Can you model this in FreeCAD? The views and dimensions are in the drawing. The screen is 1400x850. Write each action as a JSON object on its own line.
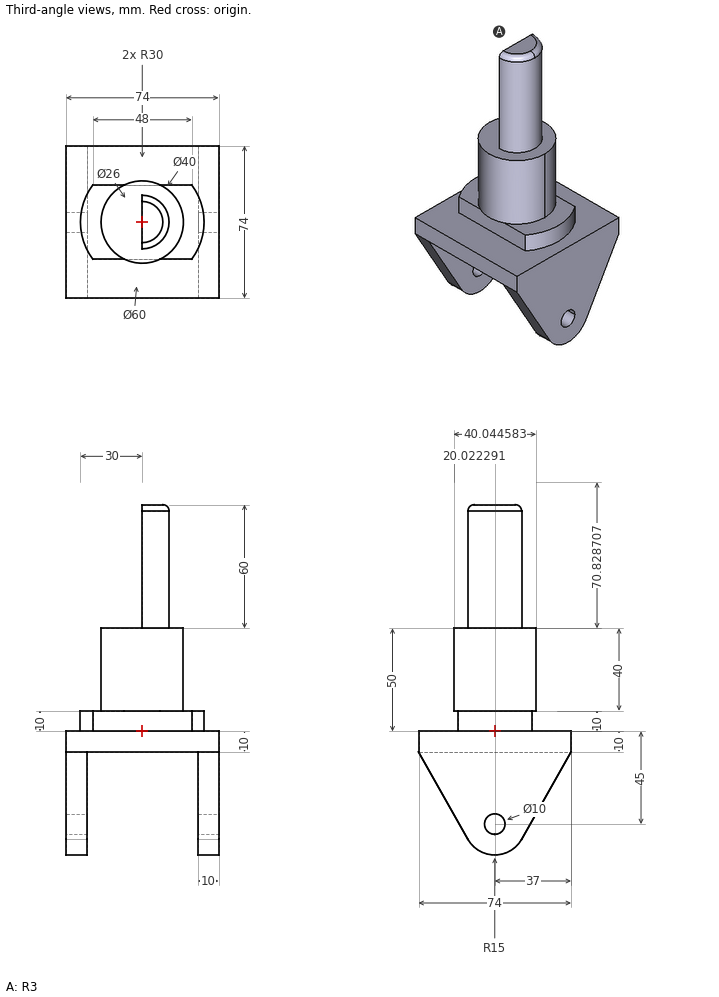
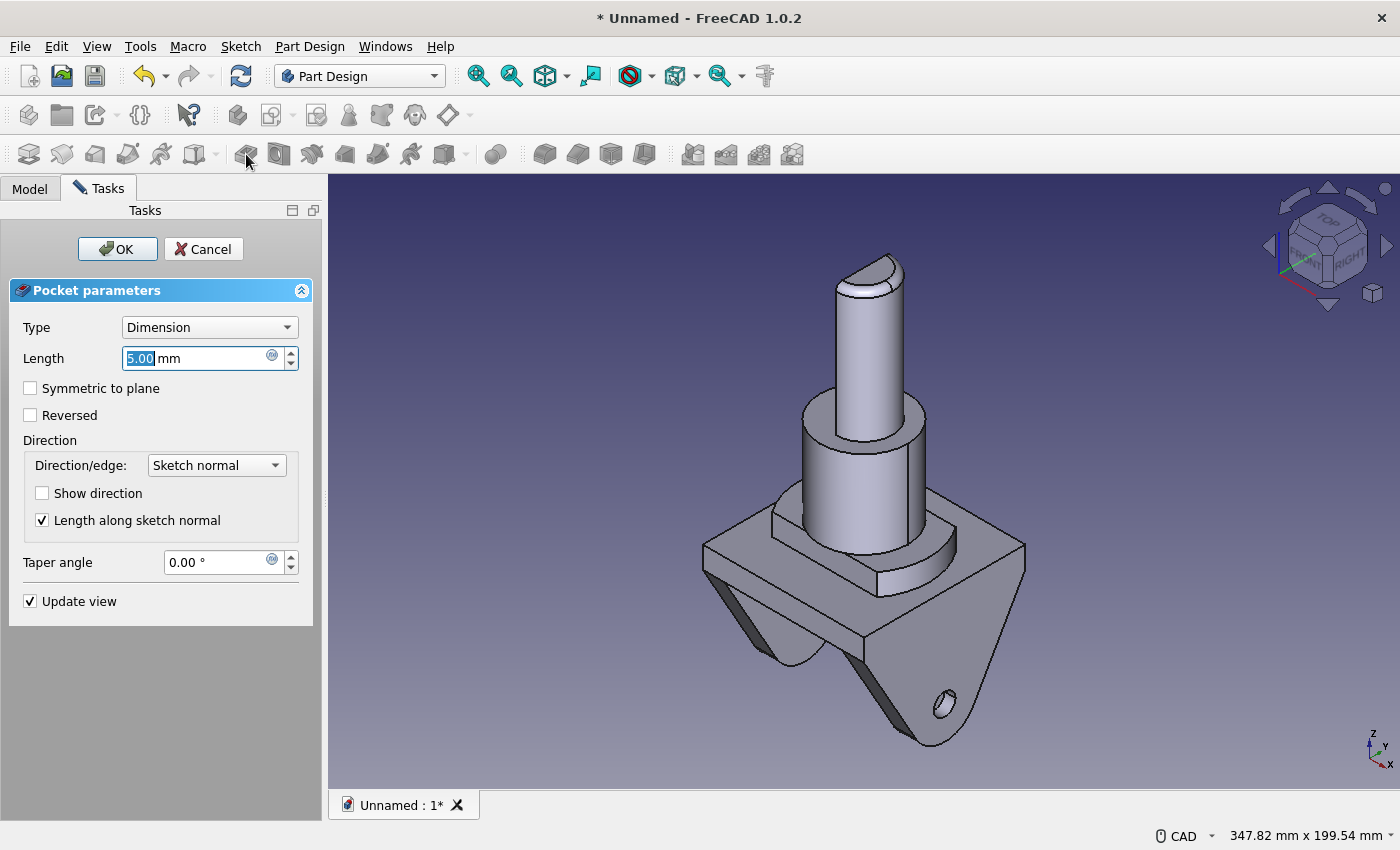
{"action": "left_click", "coordinate": [210, 328]}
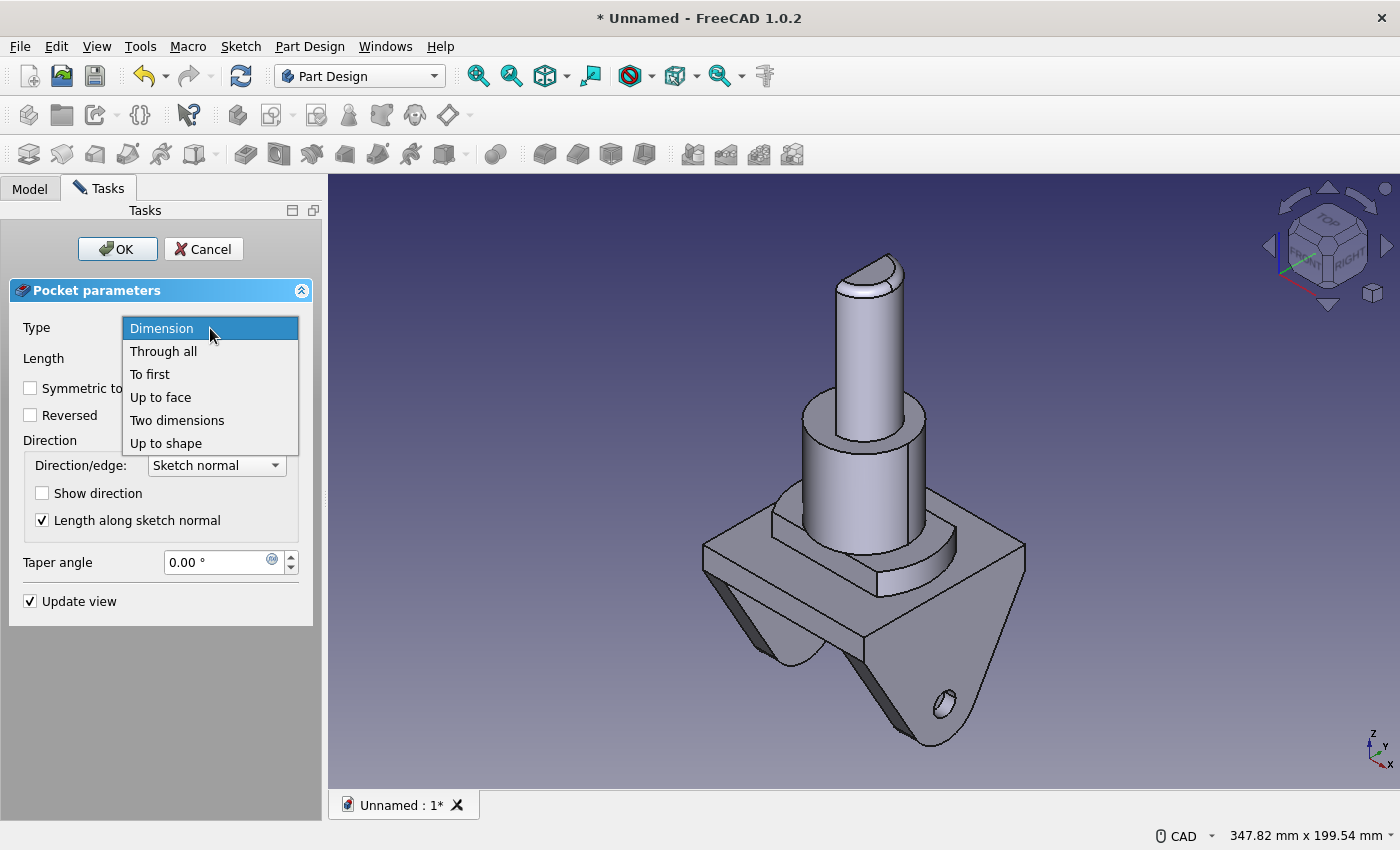
{"action": "left_click", "coordinate": [208, 352]}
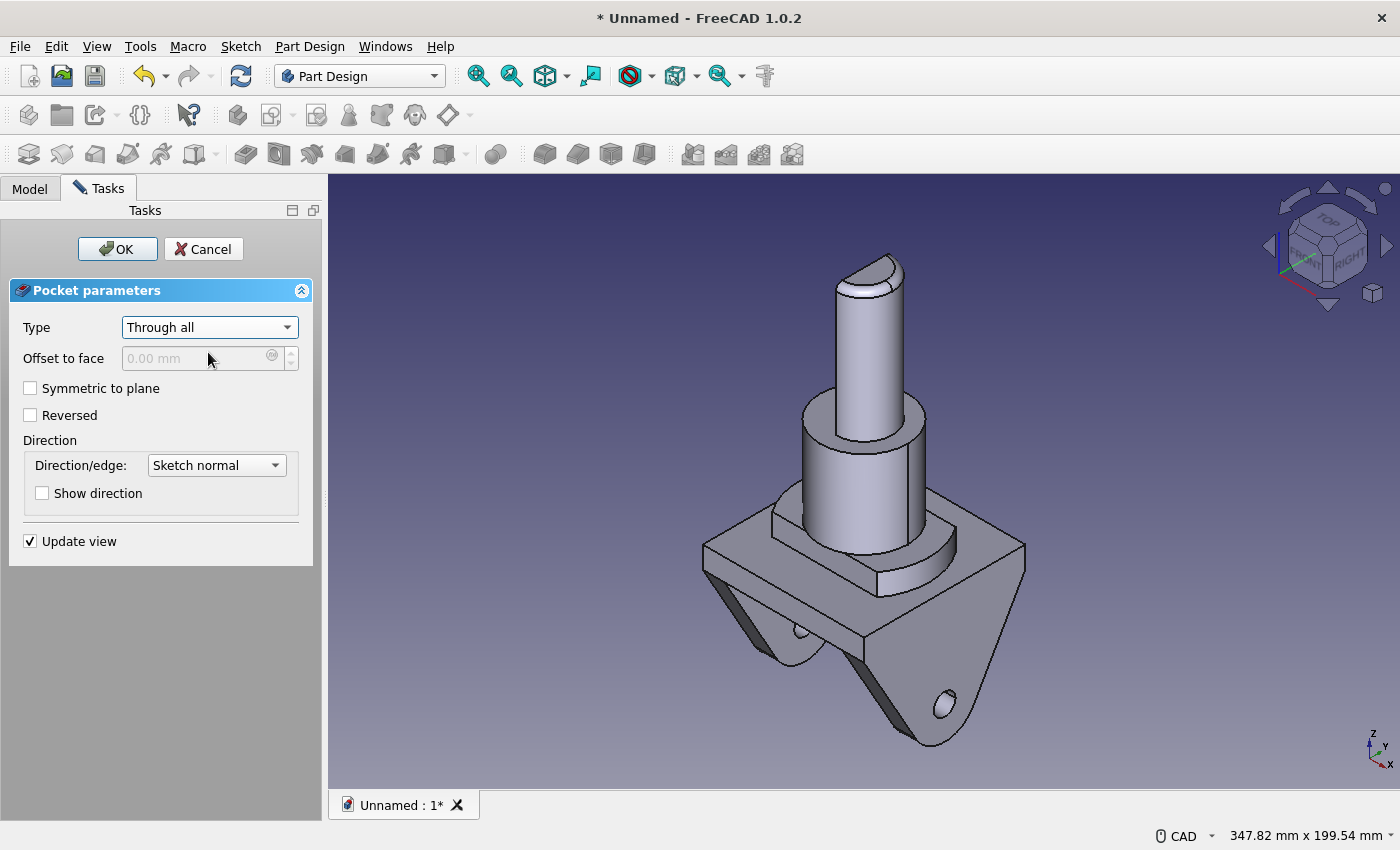
{"action": "left_click", "coordinate": [118, 249]}